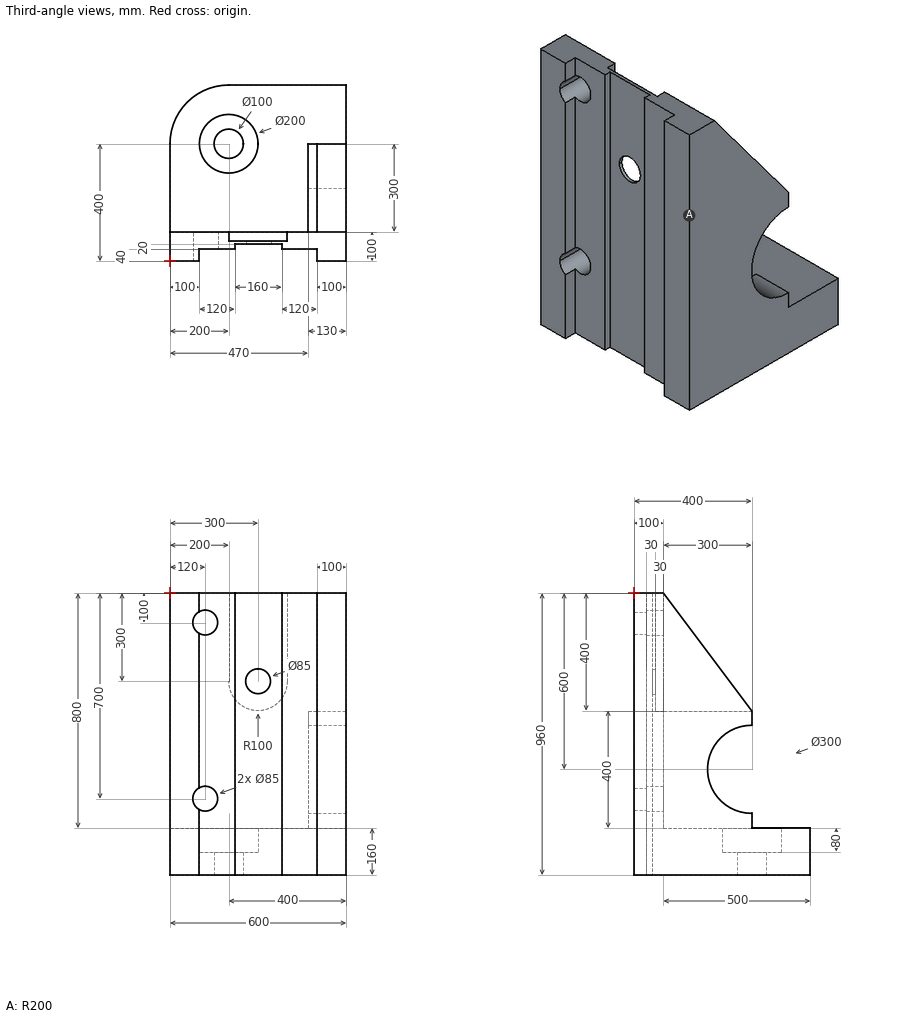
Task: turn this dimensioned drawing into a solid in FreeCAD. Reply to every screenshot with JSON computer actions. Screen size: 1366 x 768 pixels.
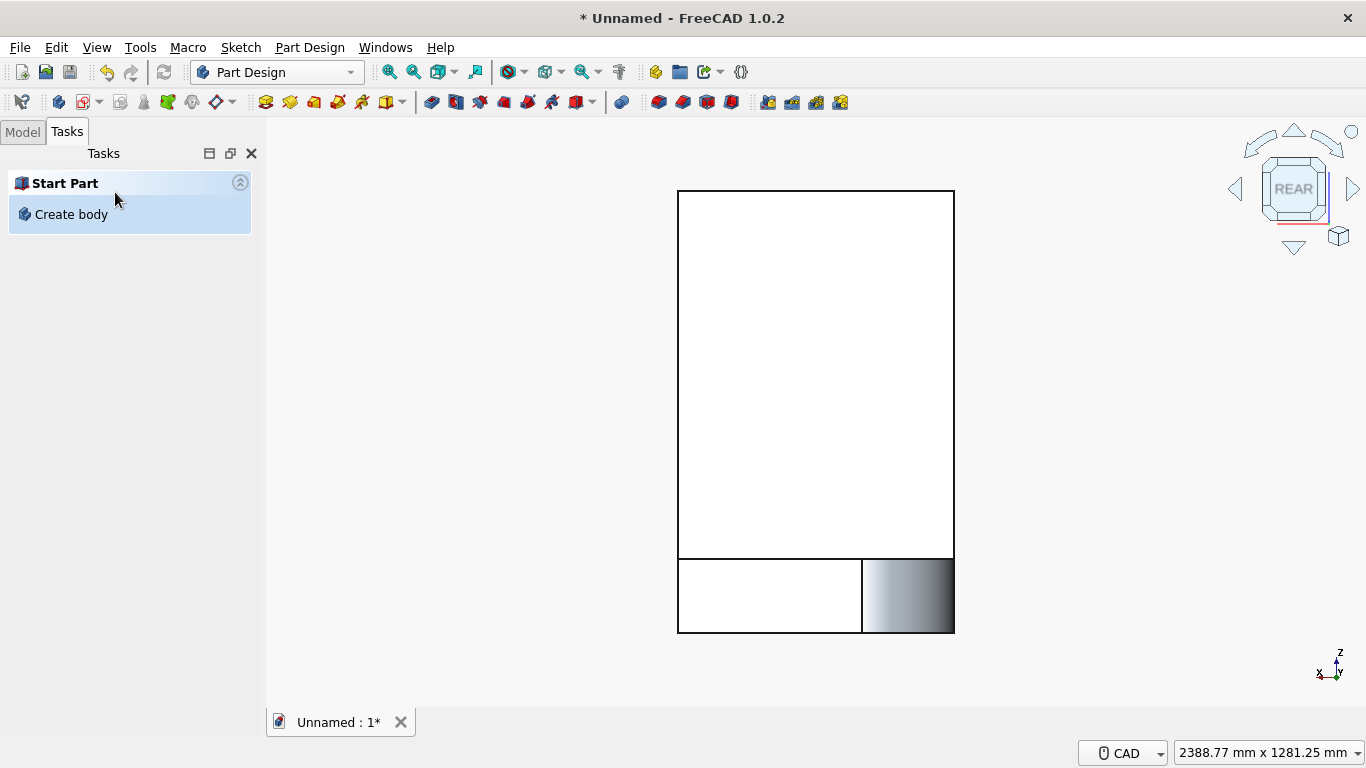
{"action": "left_click", "coordinate": [816, 374]}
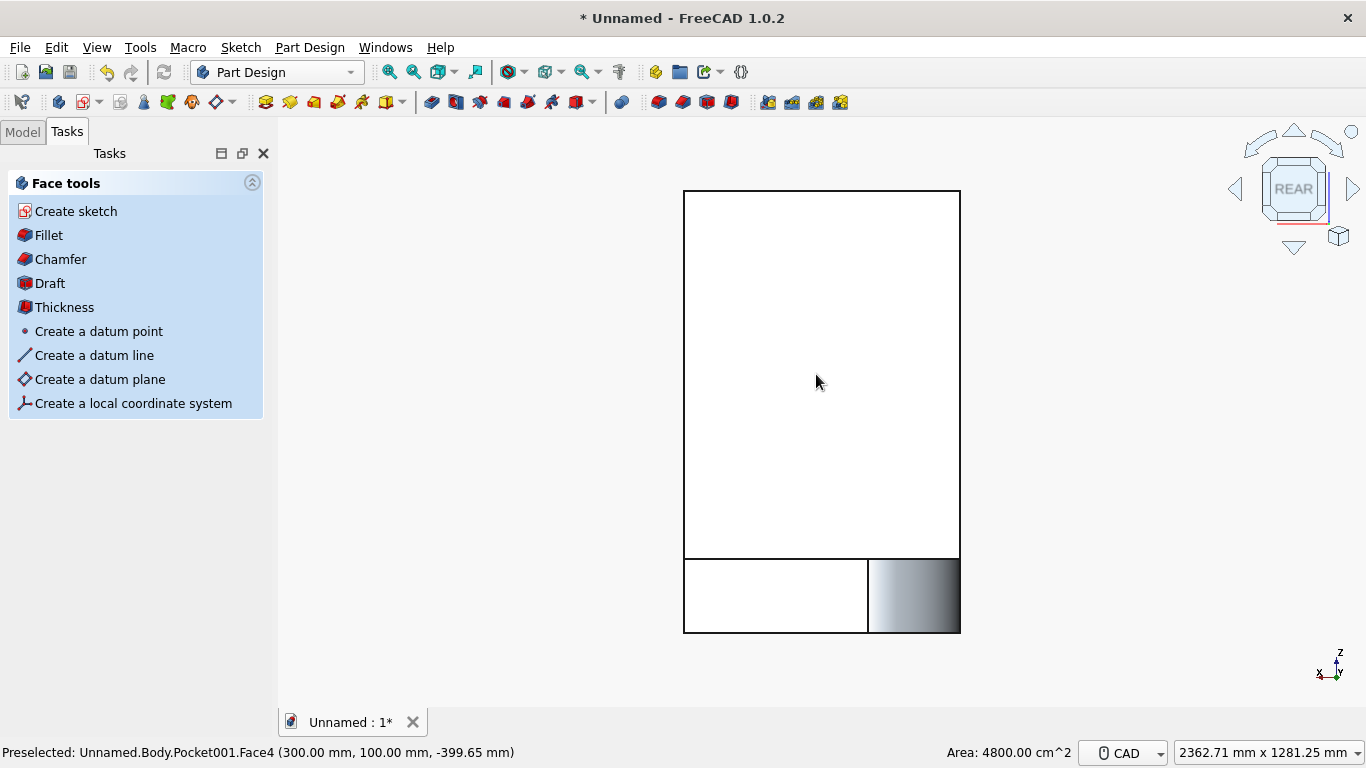
{"action": "left_click", "coordinate": [84, 102]}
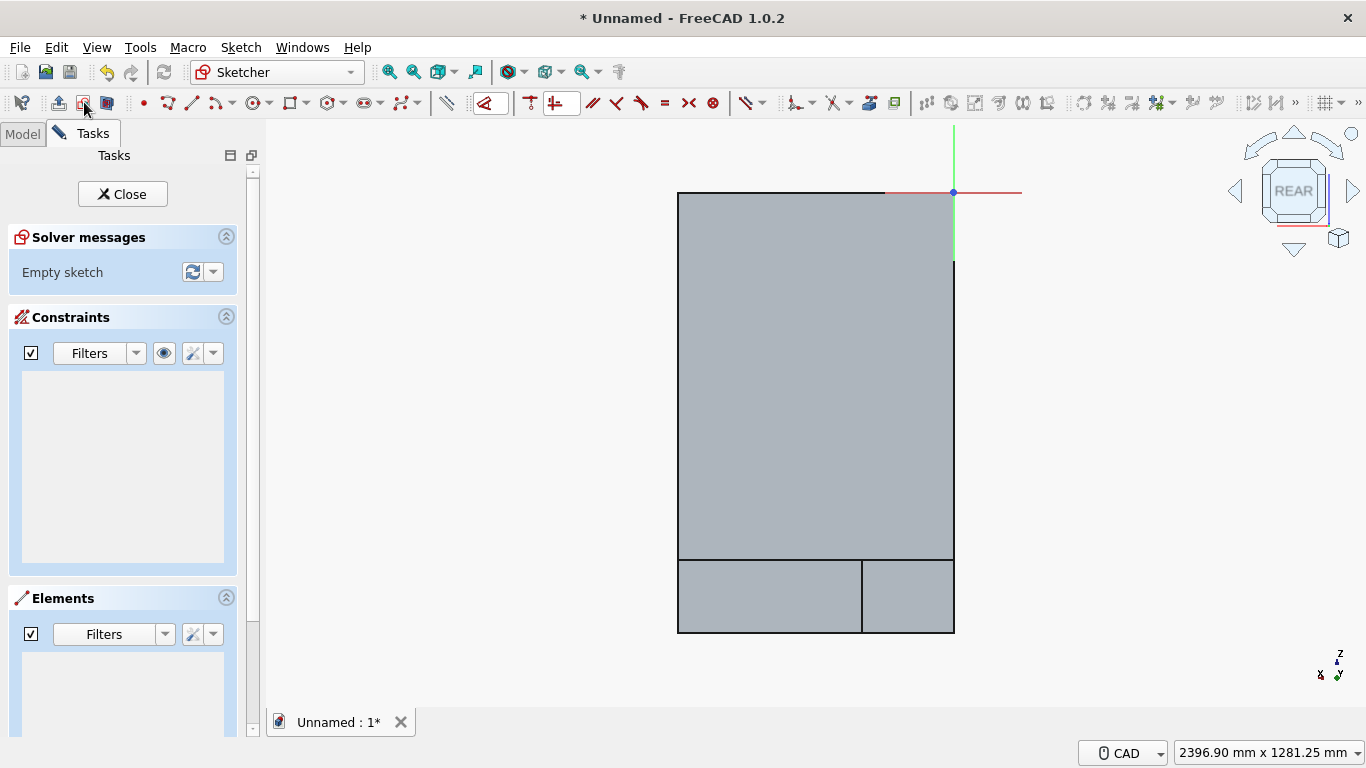
{"action": "key", "text": "g c"}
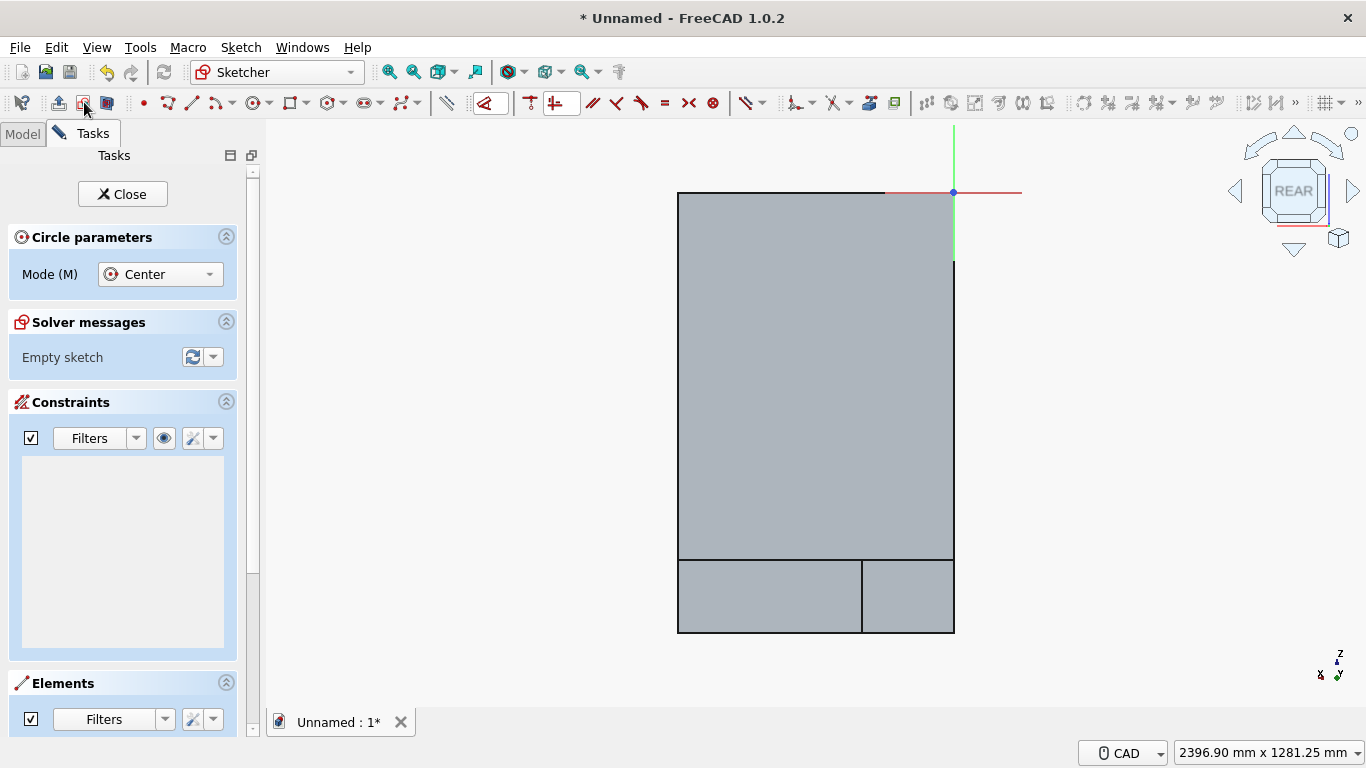
{"action": "left_click", "coordinate": [899, 514]}
{"action": "left_click", "coordinate": [912, 500]}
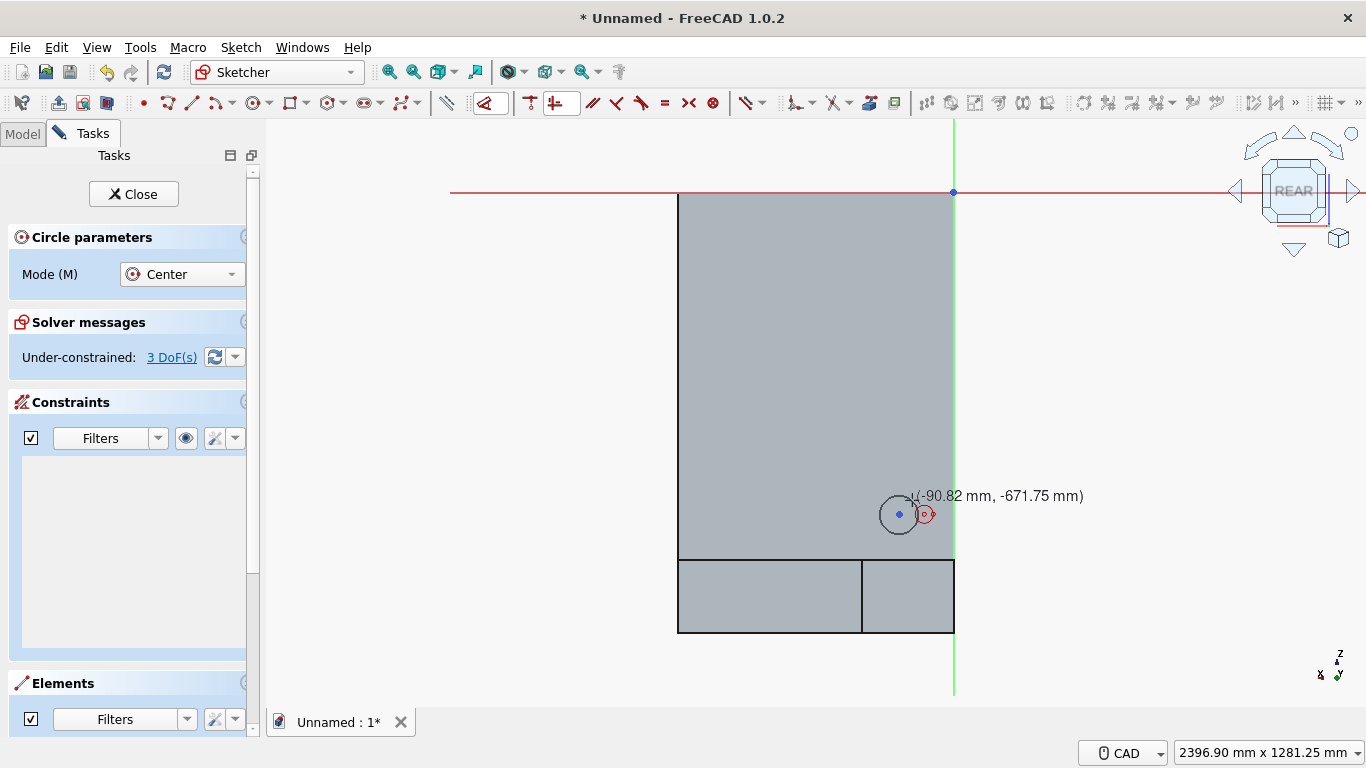
{"action": "left_click", "coordinate": [899, 239]}
{"action": "left_click", "coordinate": [912, 225]}
{"action": "key", "text": "Escape"}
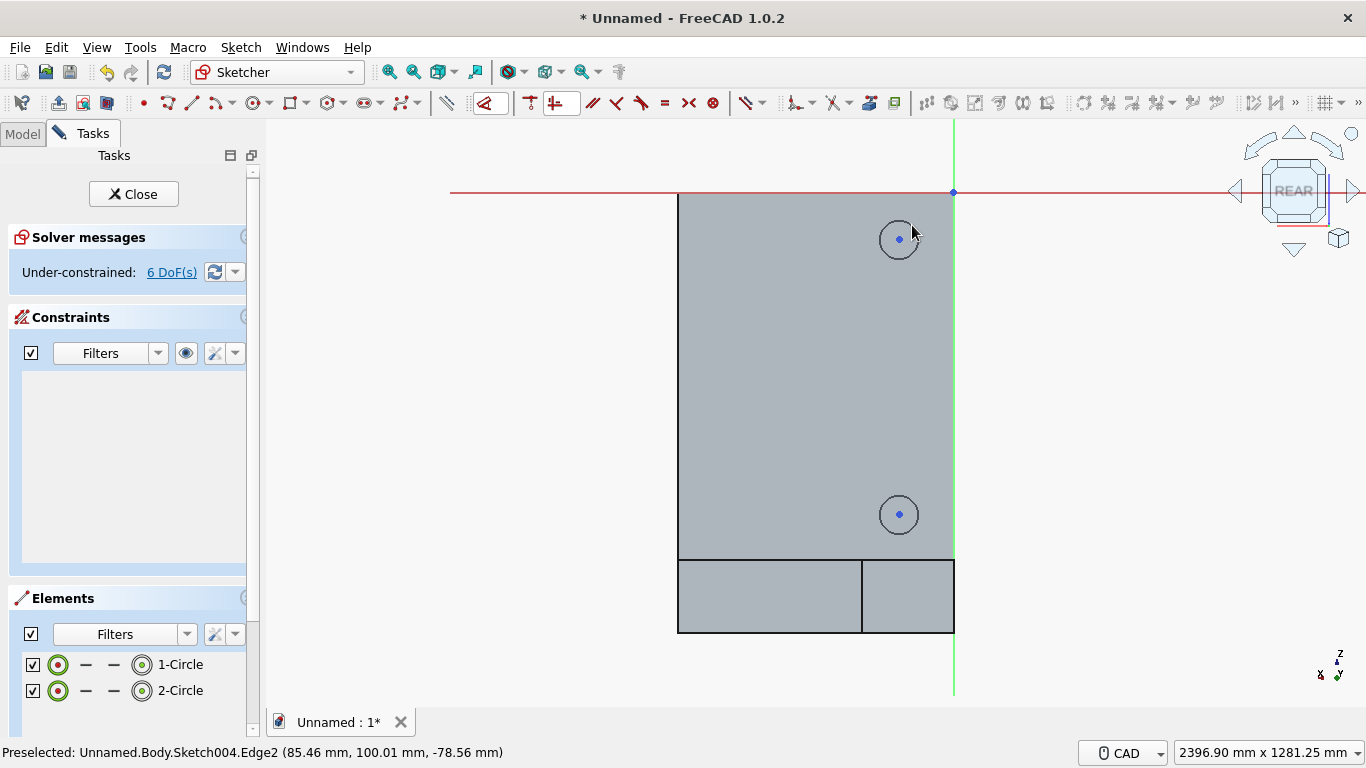
{"action": "left_click", "coordinate": [912, 501]}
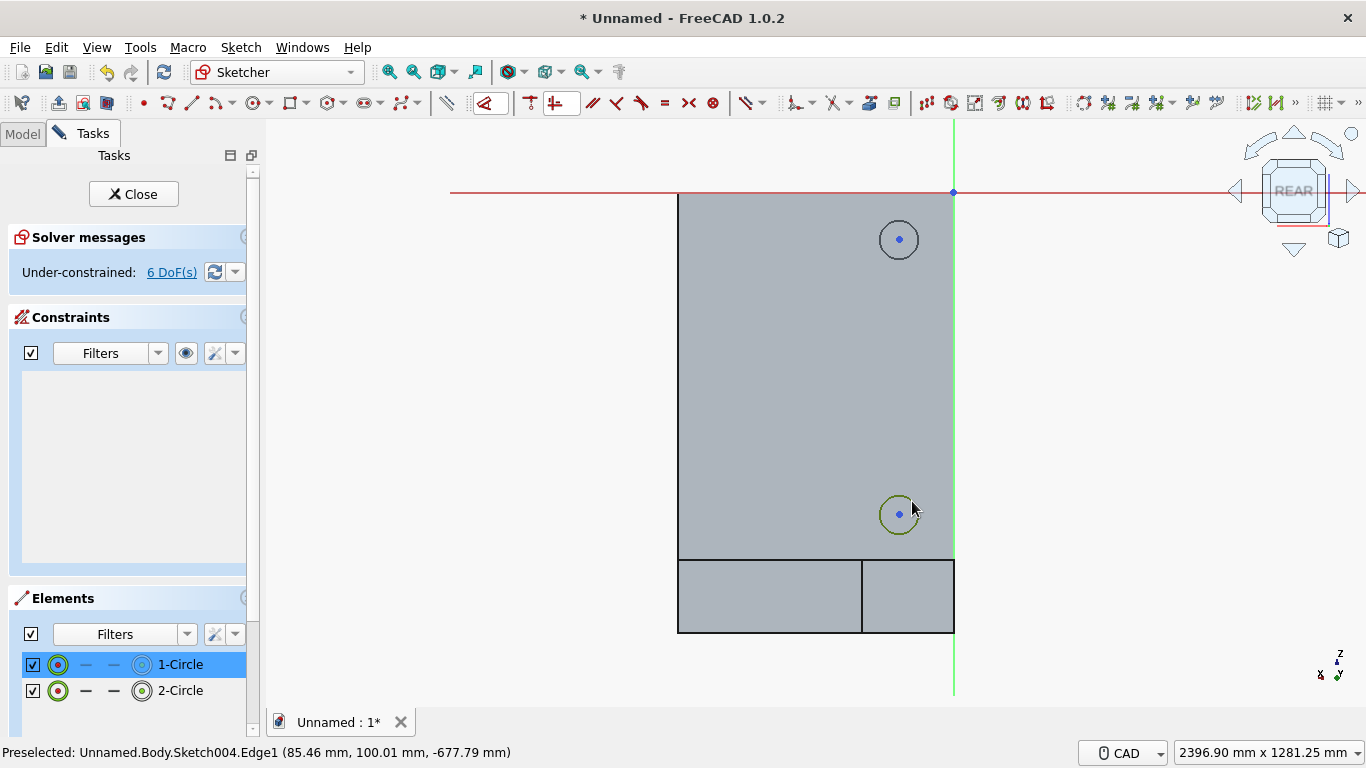
{"action": "left_click", "coordinate": [912, 226]}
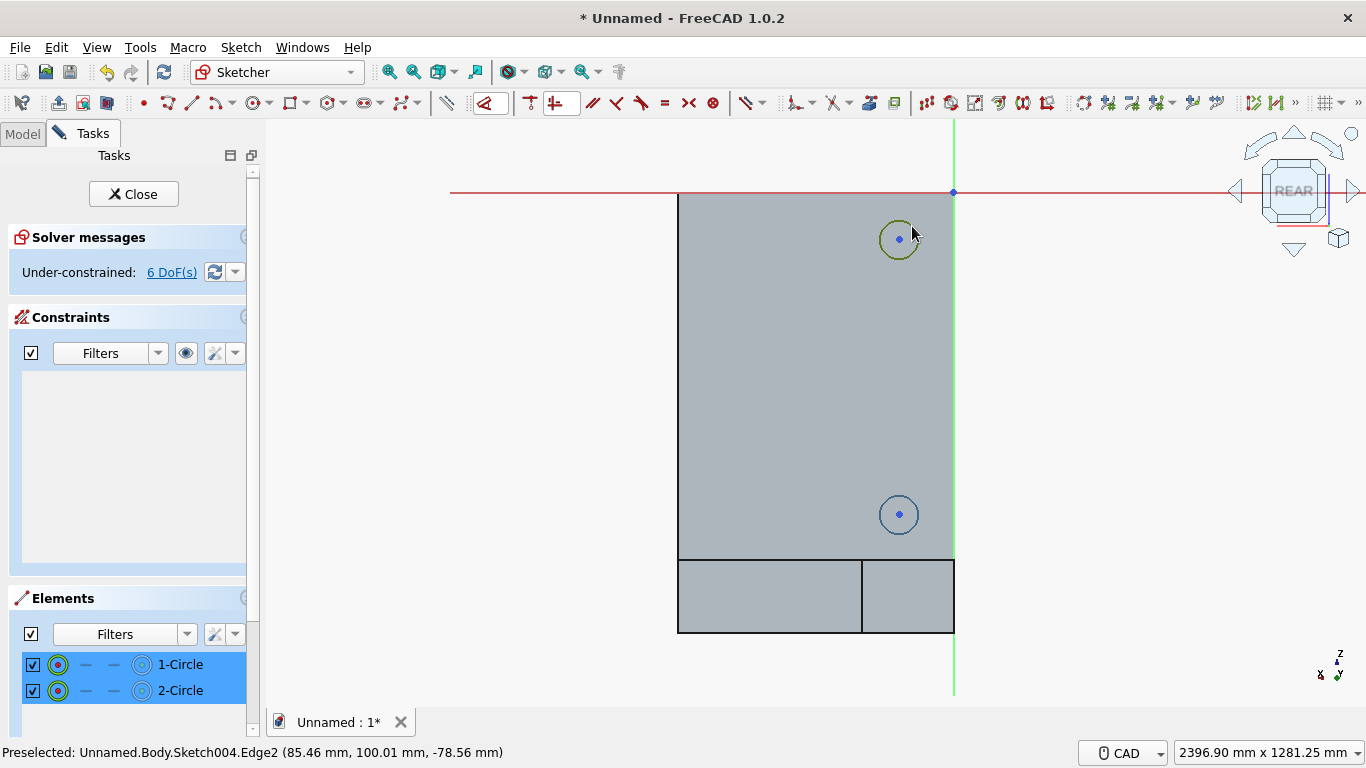
{"action": "left_click", "coordinate": [666, 104]}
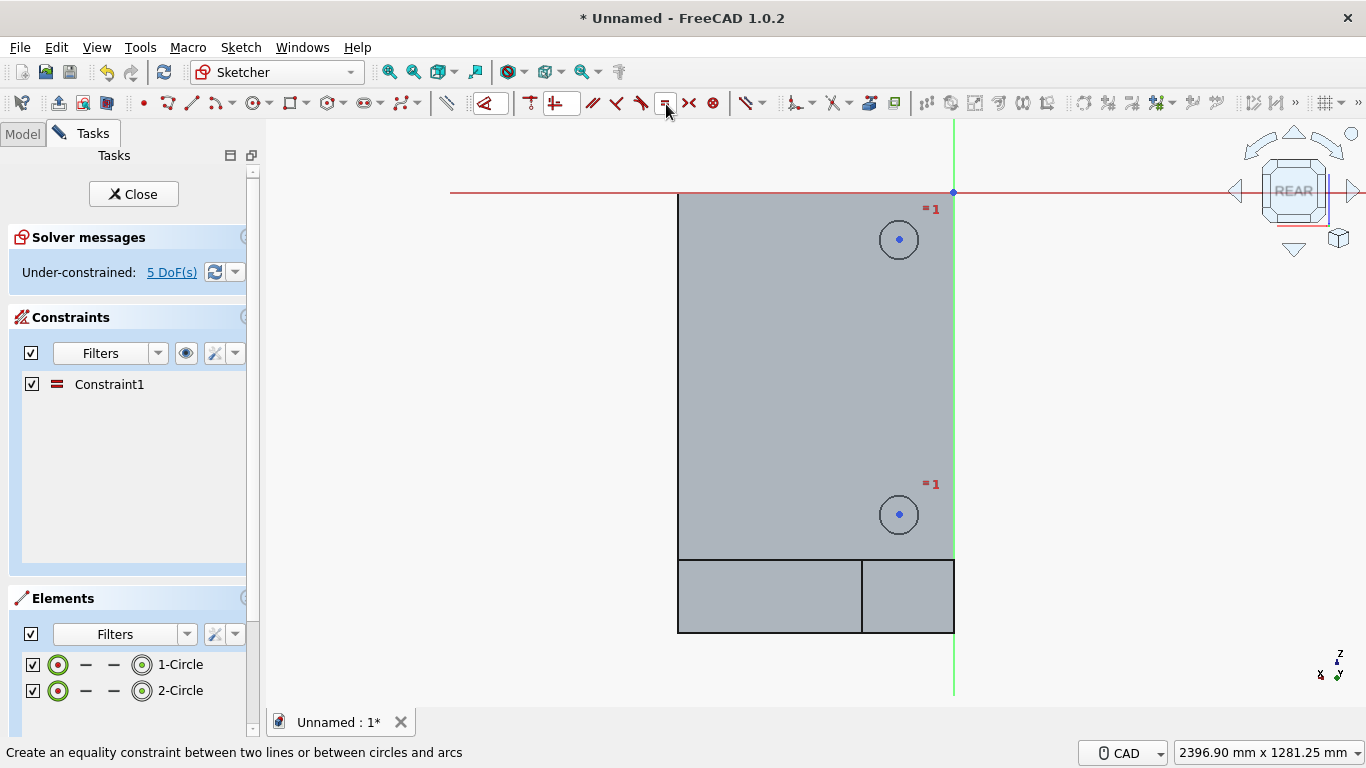
{"action": "left_click", "coordinate": [899, 515]}